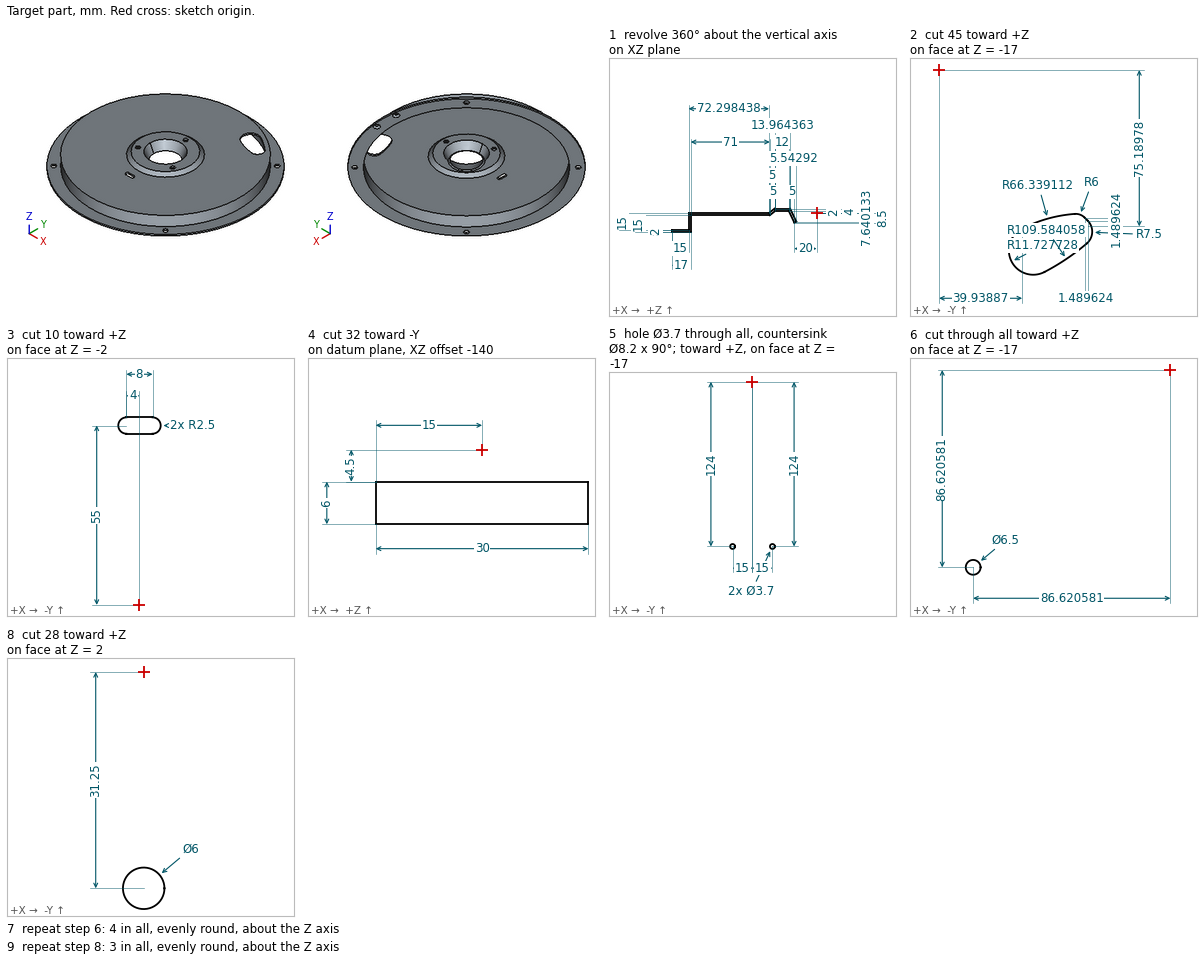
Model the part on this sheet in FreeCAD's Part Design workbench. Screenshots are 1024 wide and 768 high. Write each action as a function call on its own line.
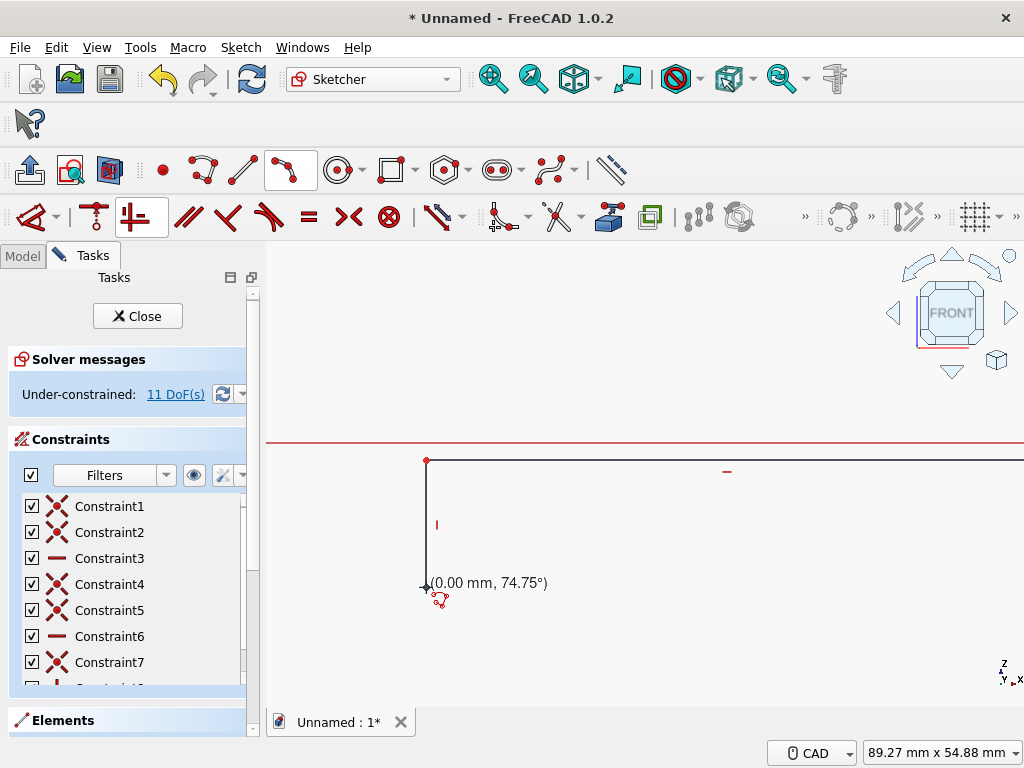
scroll(427, 460, down, 5)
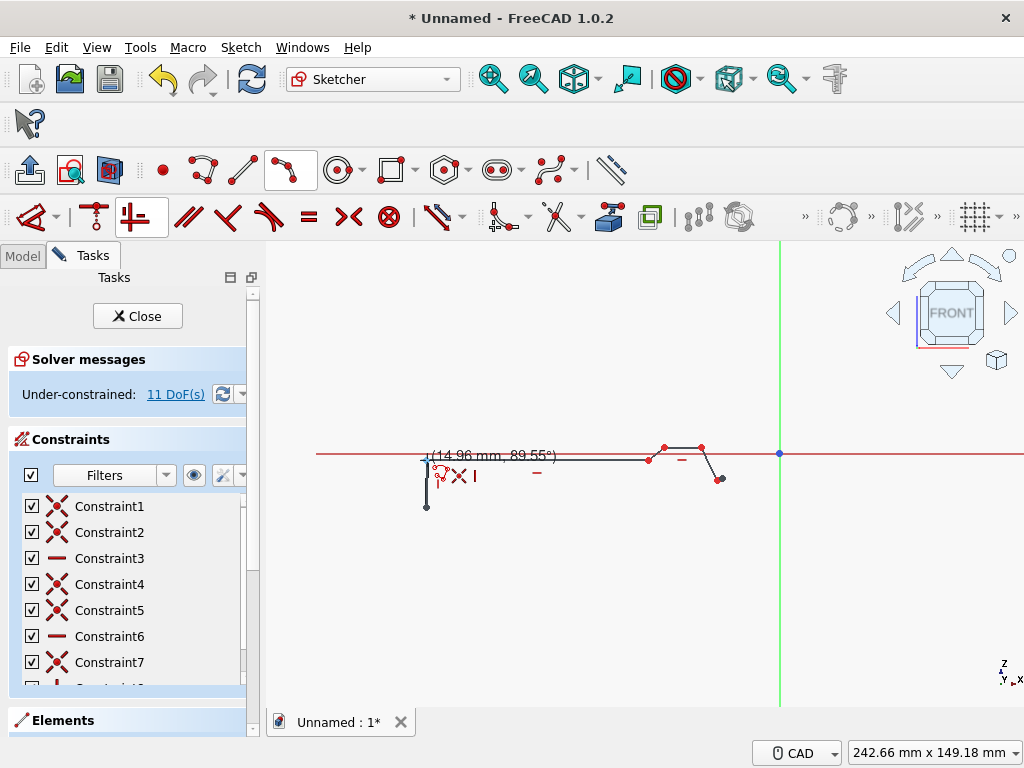
click(374, 507)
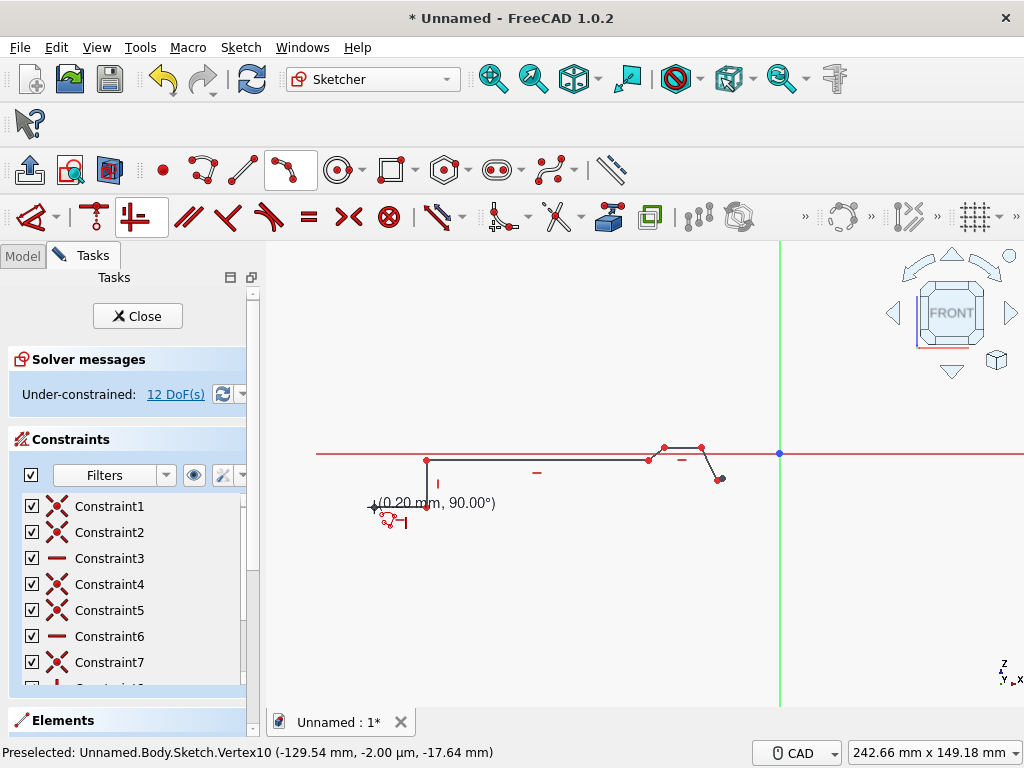
scroll(374, 501, up, 5)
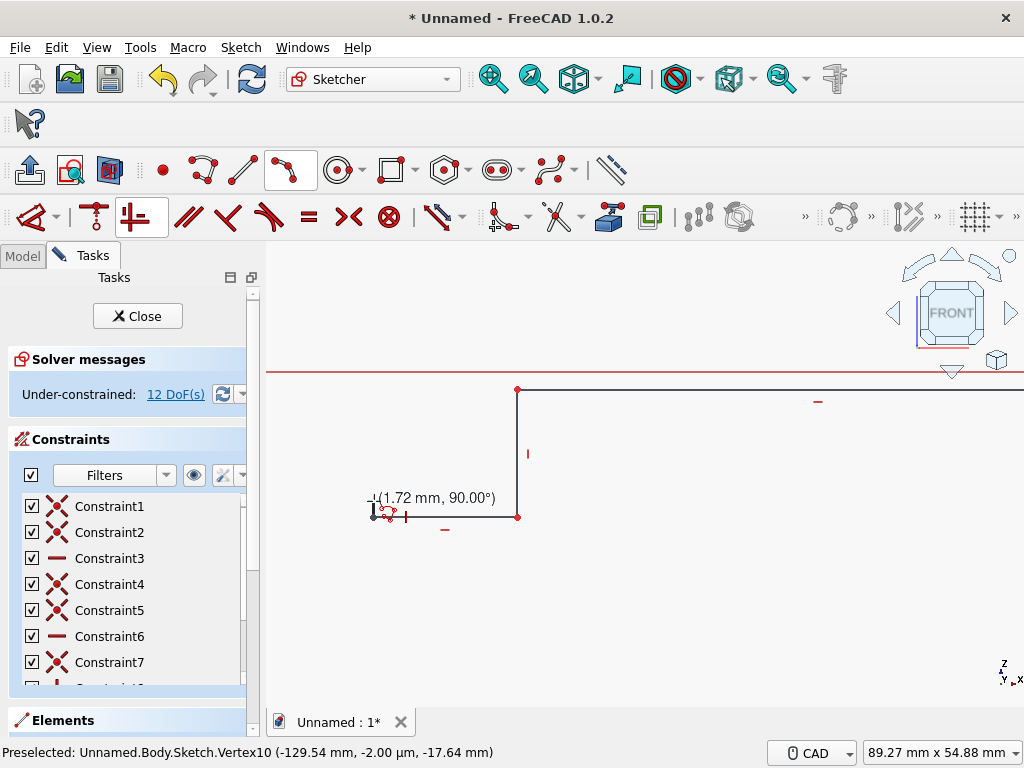
click(374, 499)
click(500, 499)
click(500, 372)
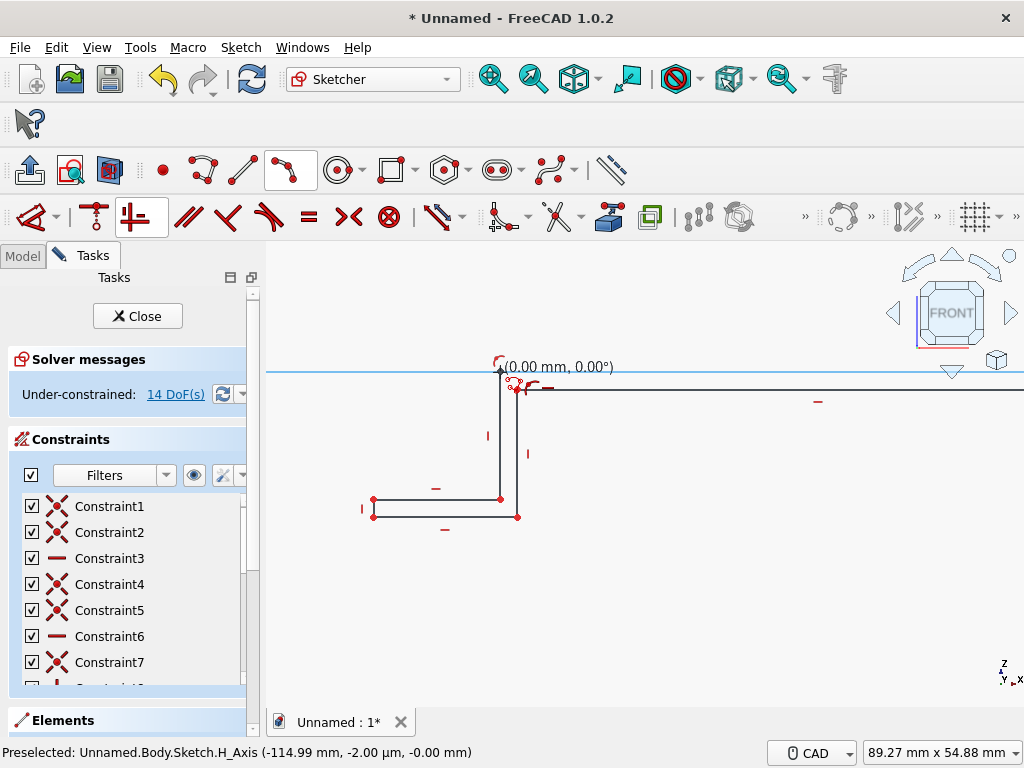
scroll(374, 501, down, 5)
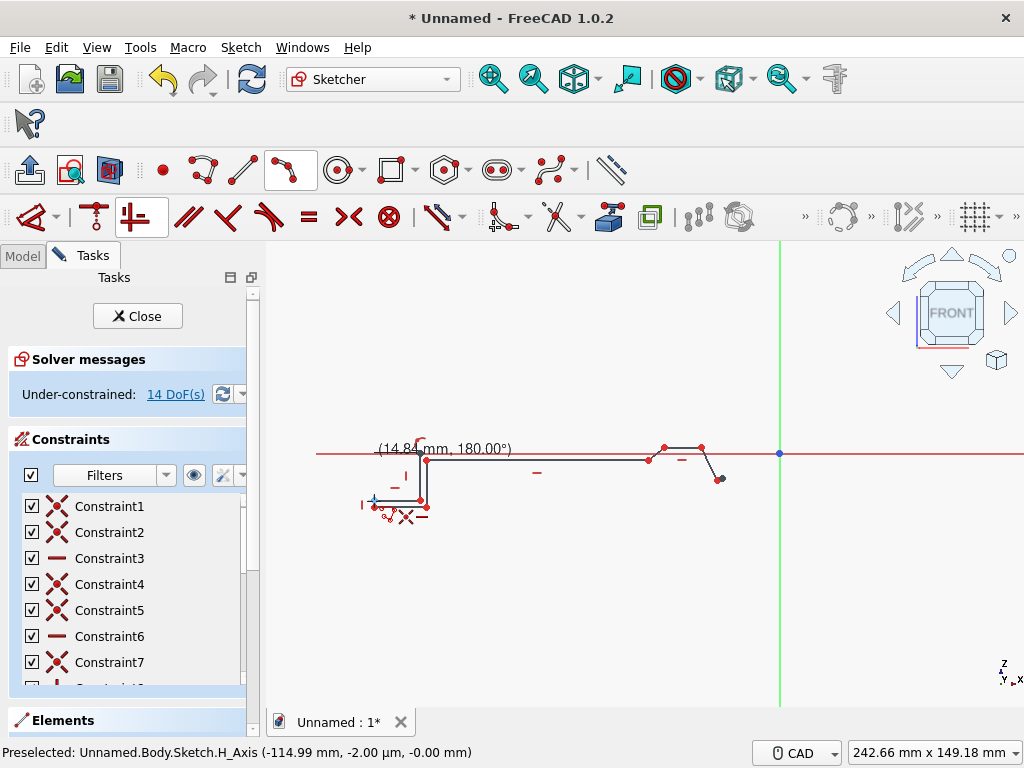
scroll(646, 454, up, 5)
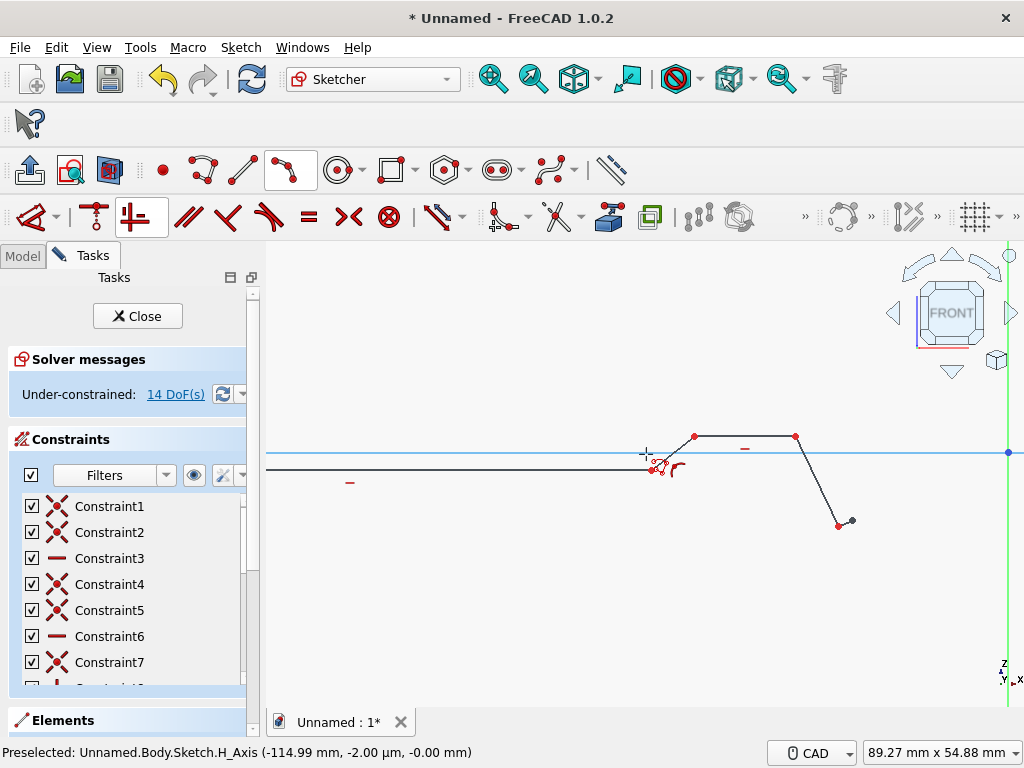
click(646, 462)
click(688, 419)
click(807, 419)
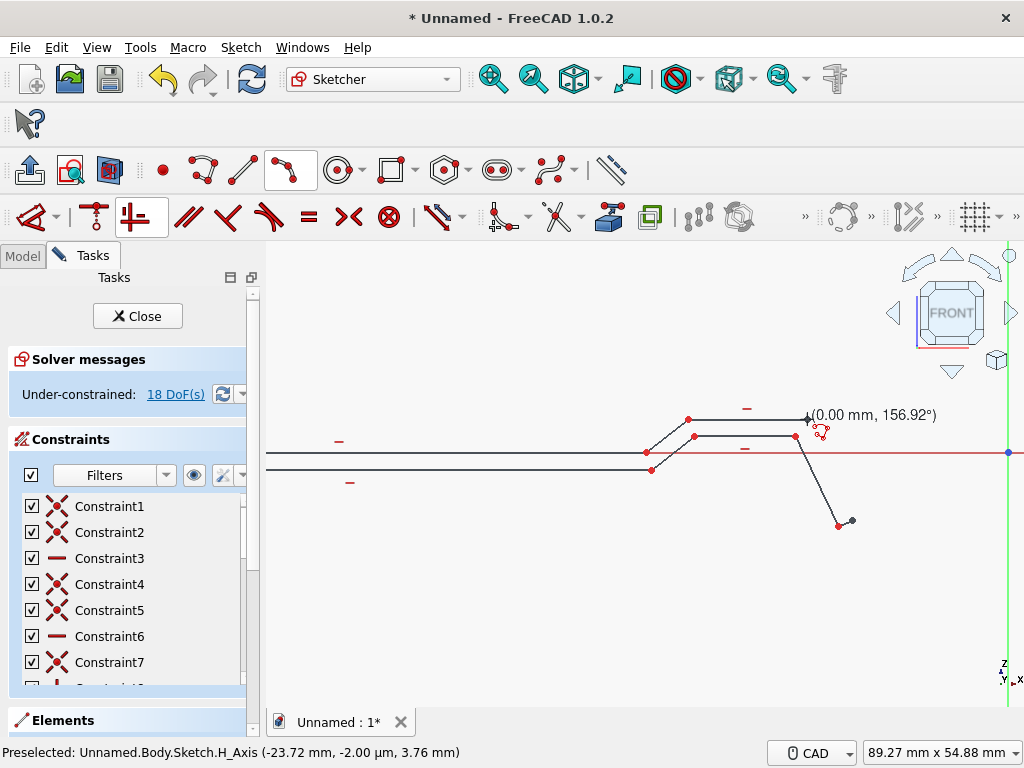
scroll(854, 518, up, 4)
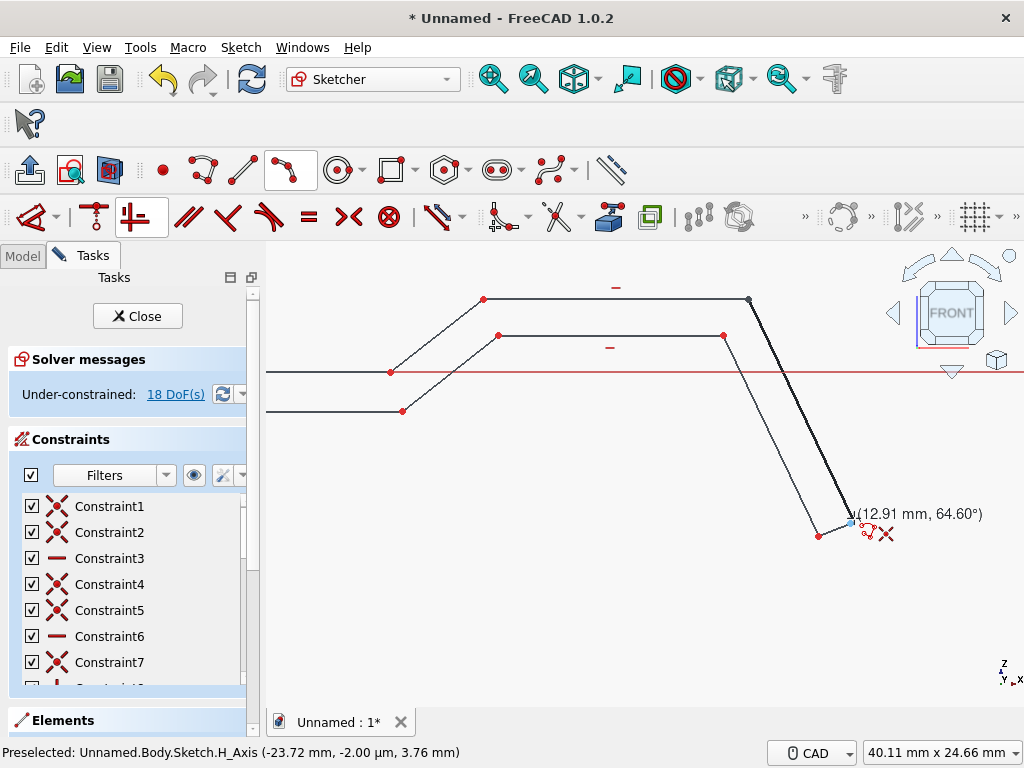
click(850, 524)
key(Escape)
key(Escape)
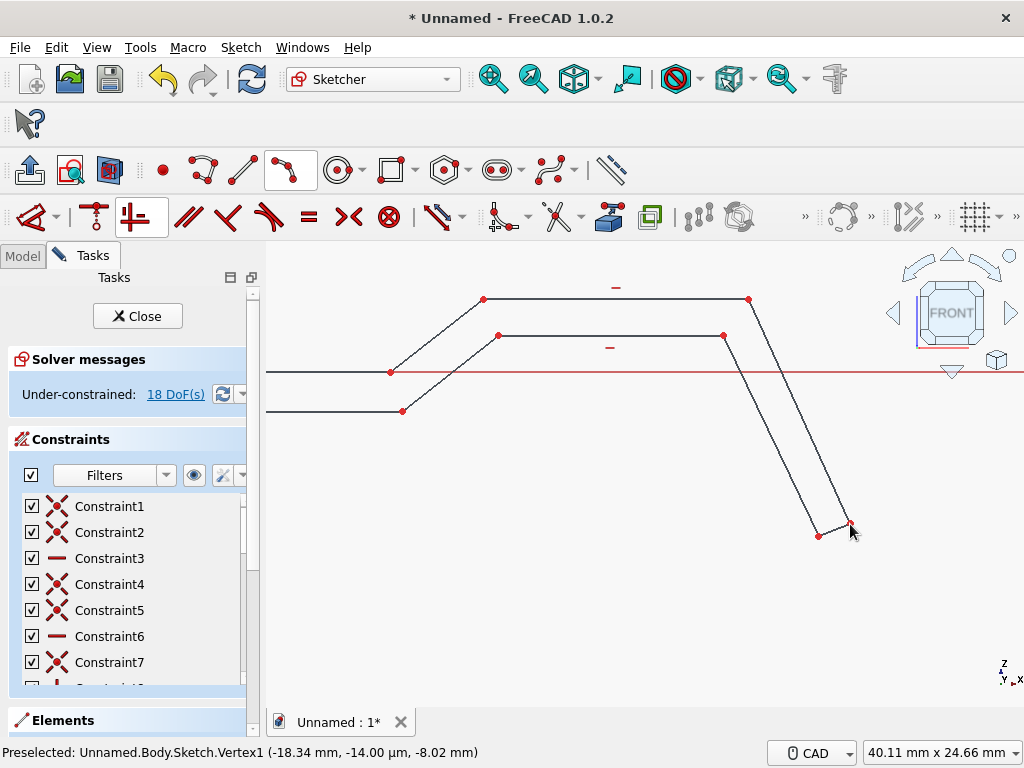
click(32, 218)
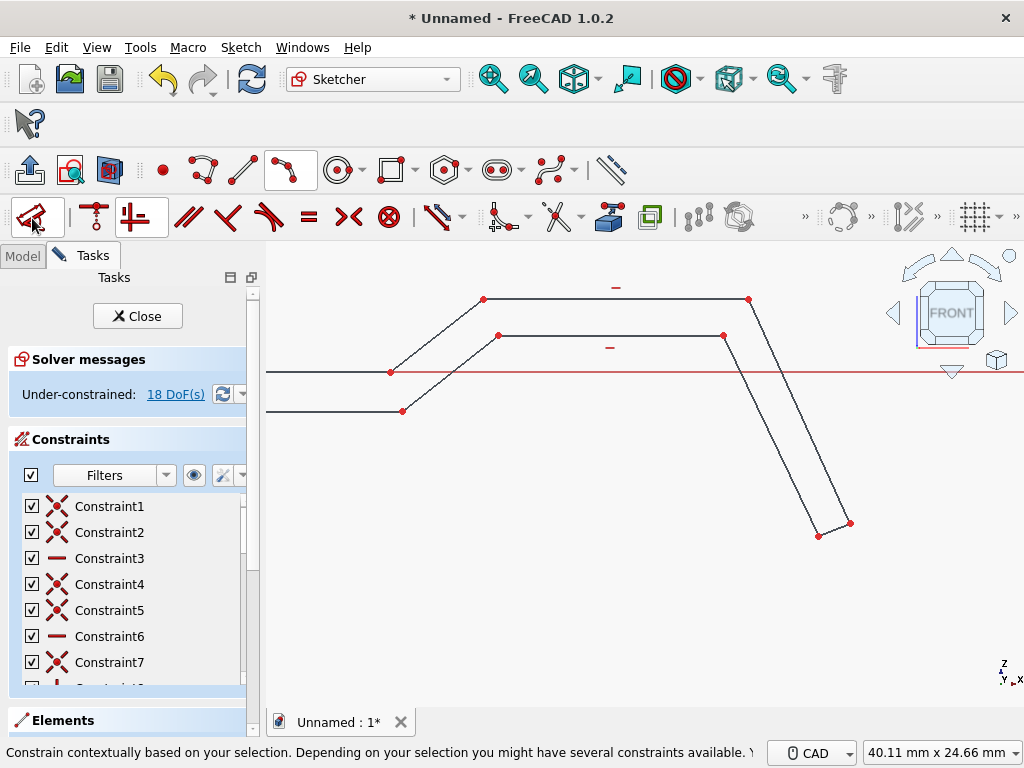
scroll(697, 470, down, 9)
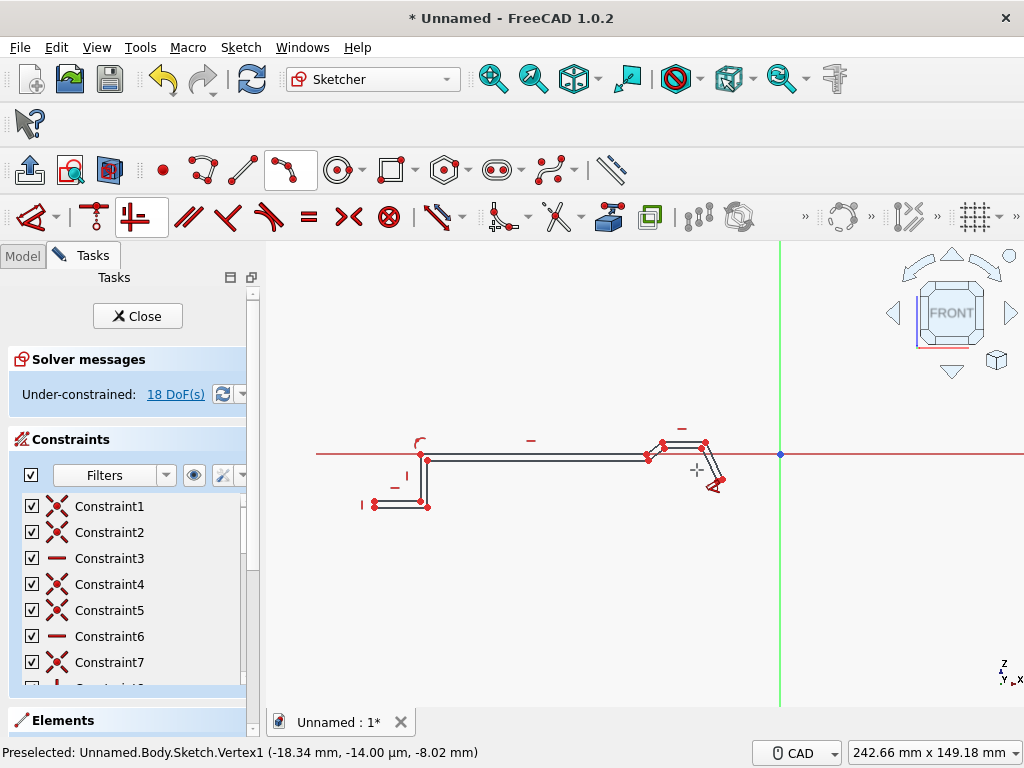
scroll(374, 506, up, 10)